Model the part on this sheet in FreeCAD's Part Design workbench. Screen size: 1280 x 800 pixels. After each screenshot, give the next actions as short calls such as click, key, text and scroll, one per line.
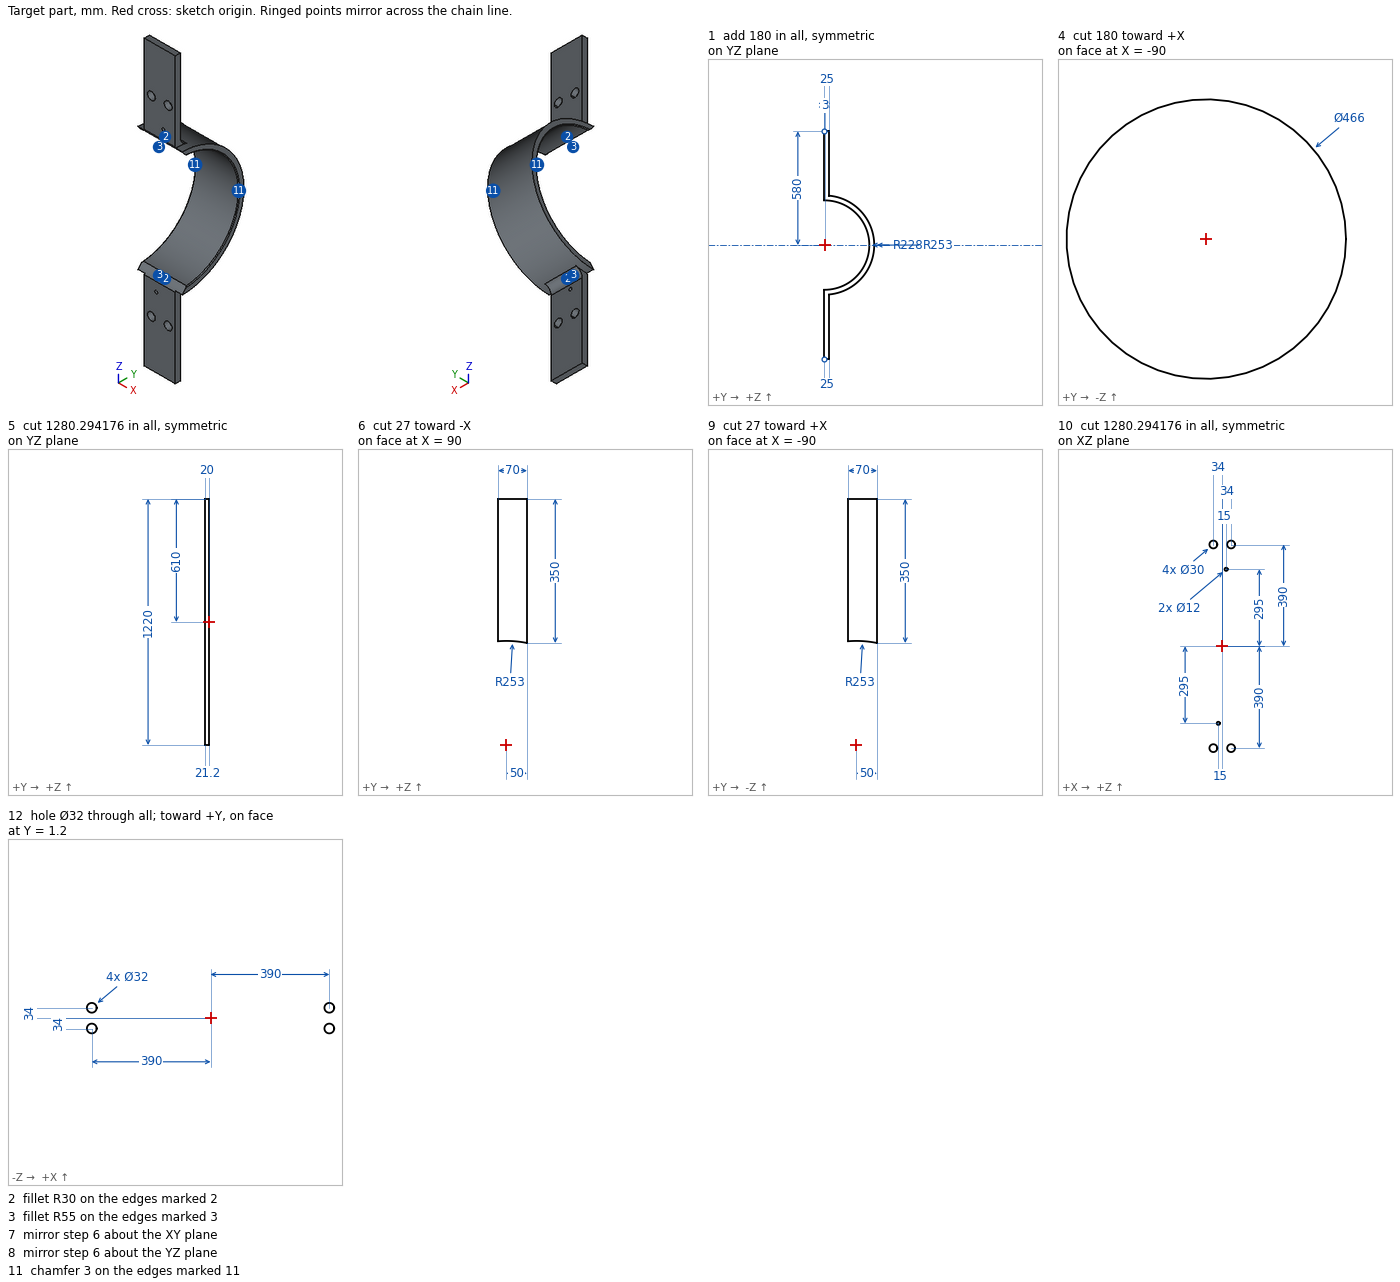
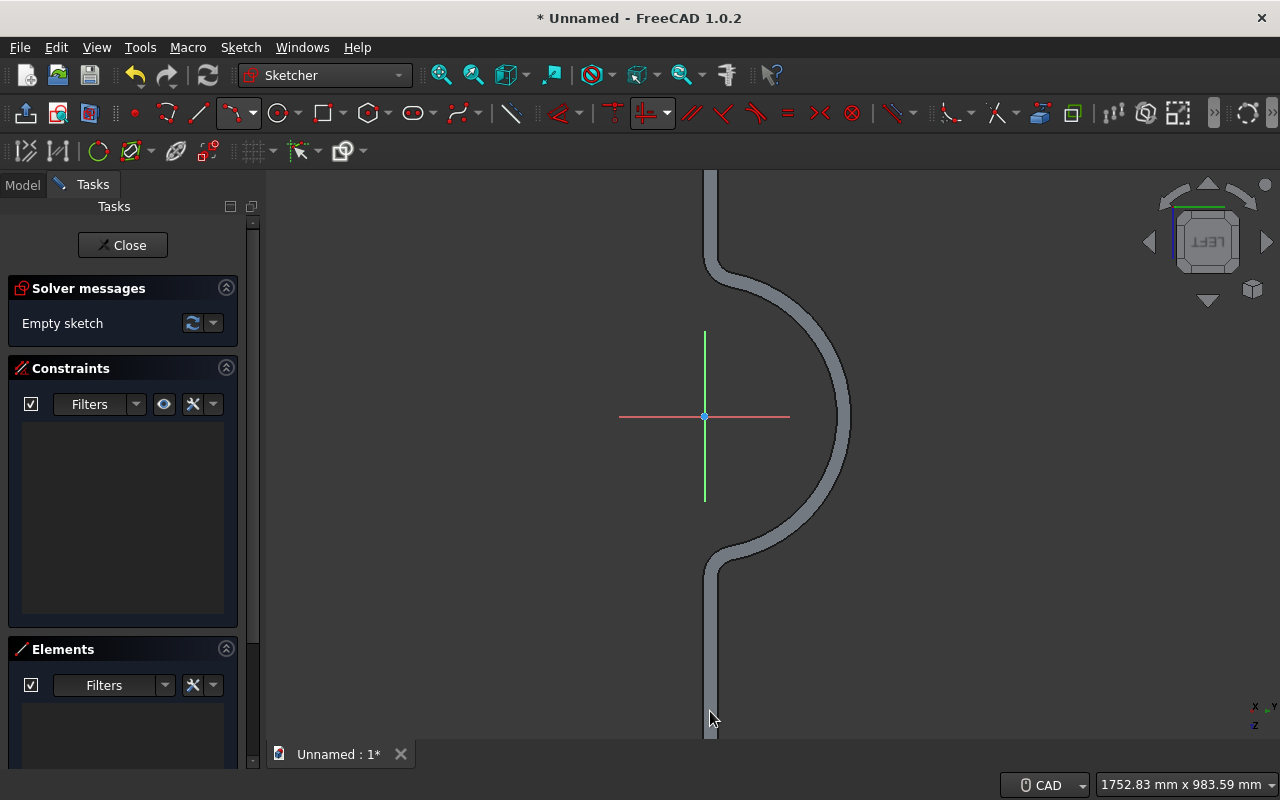
click(278, 114)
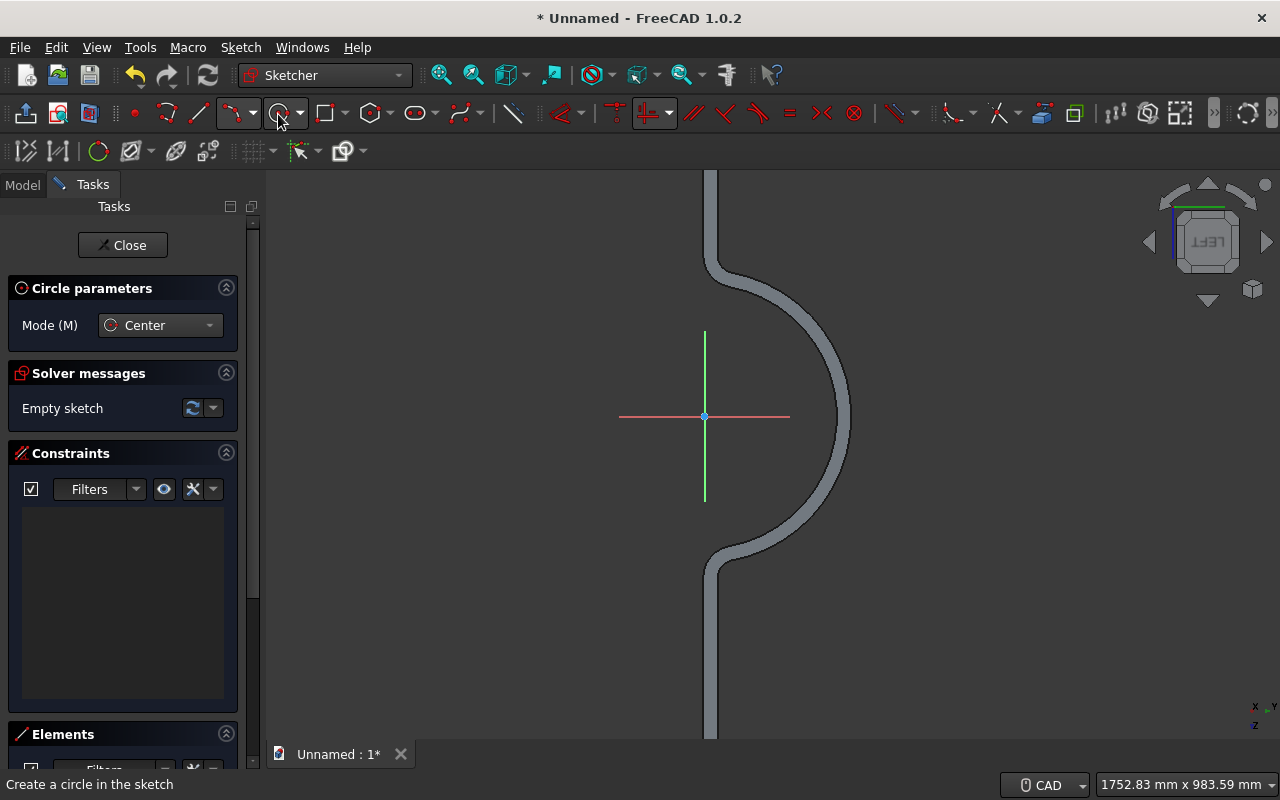
click(705, 417)
move(800, 321)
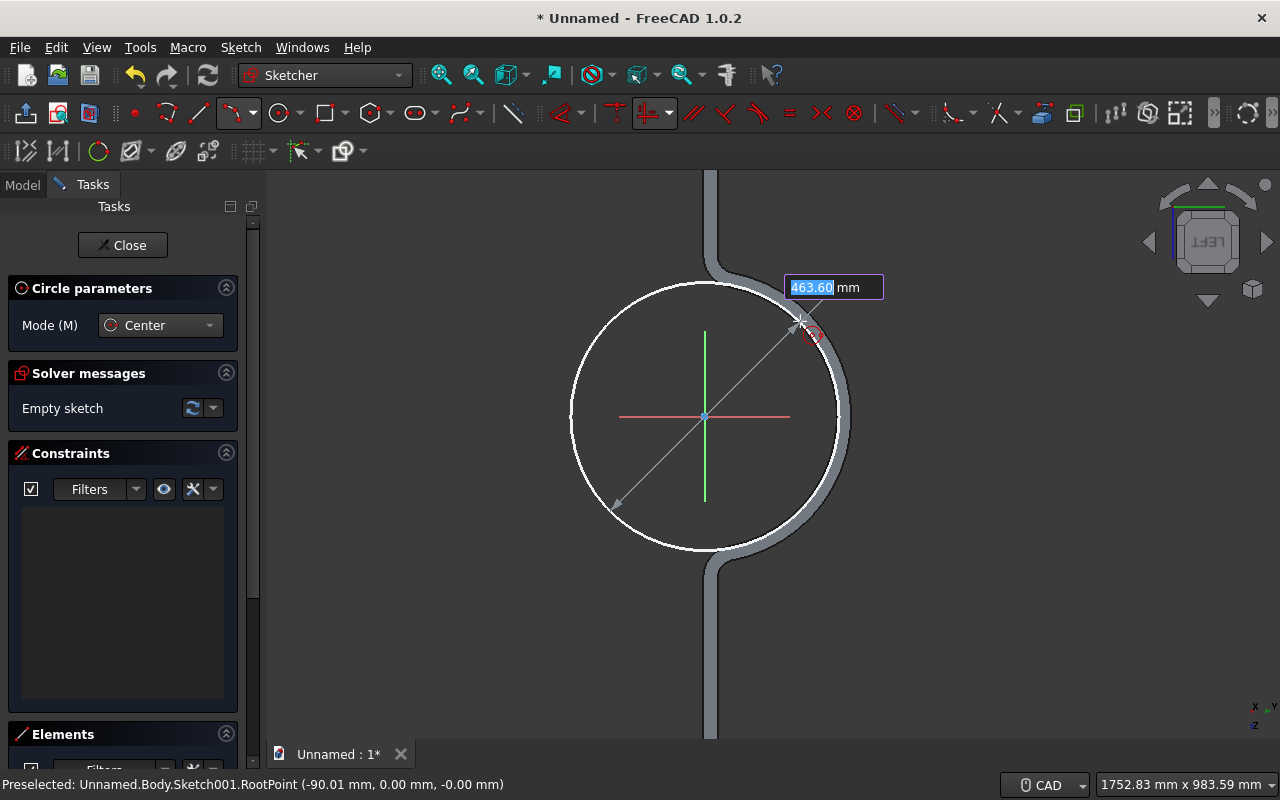
text(466)
key(Return)
key(Escape)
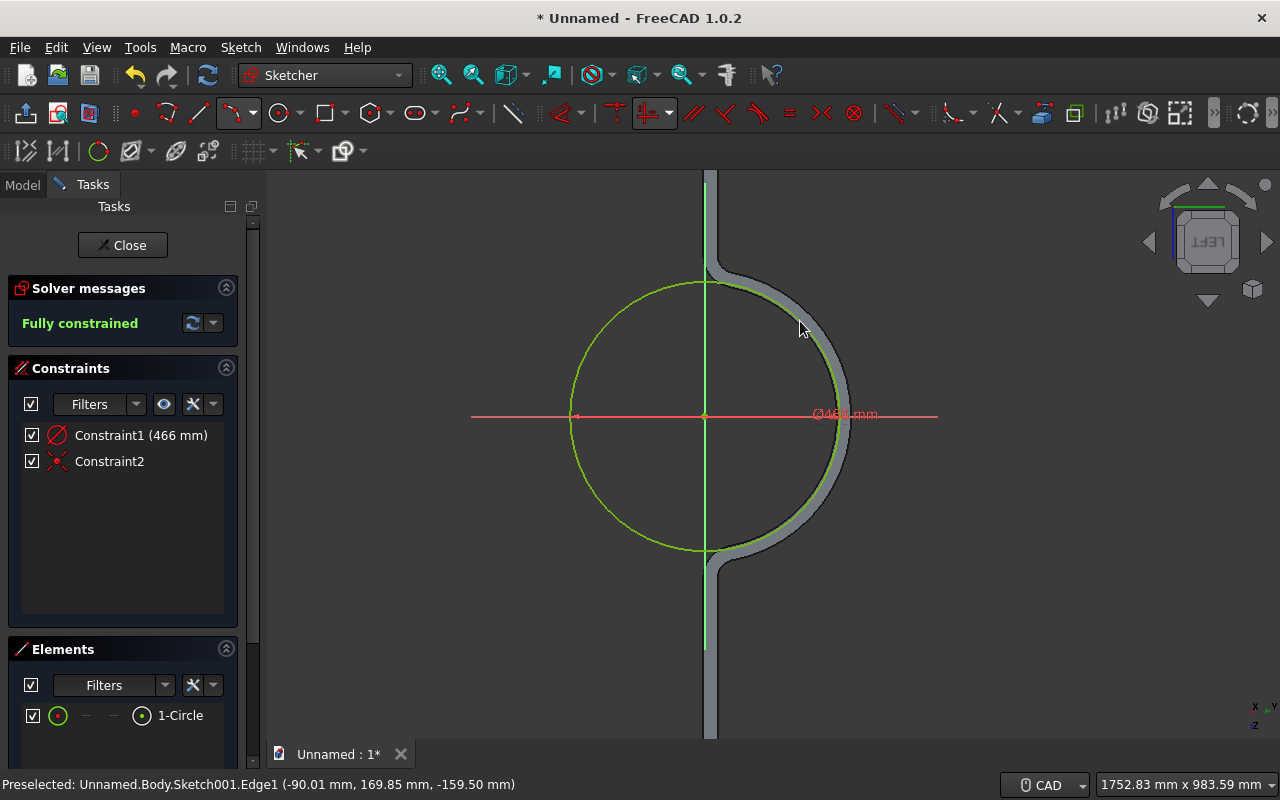
click(123, 245)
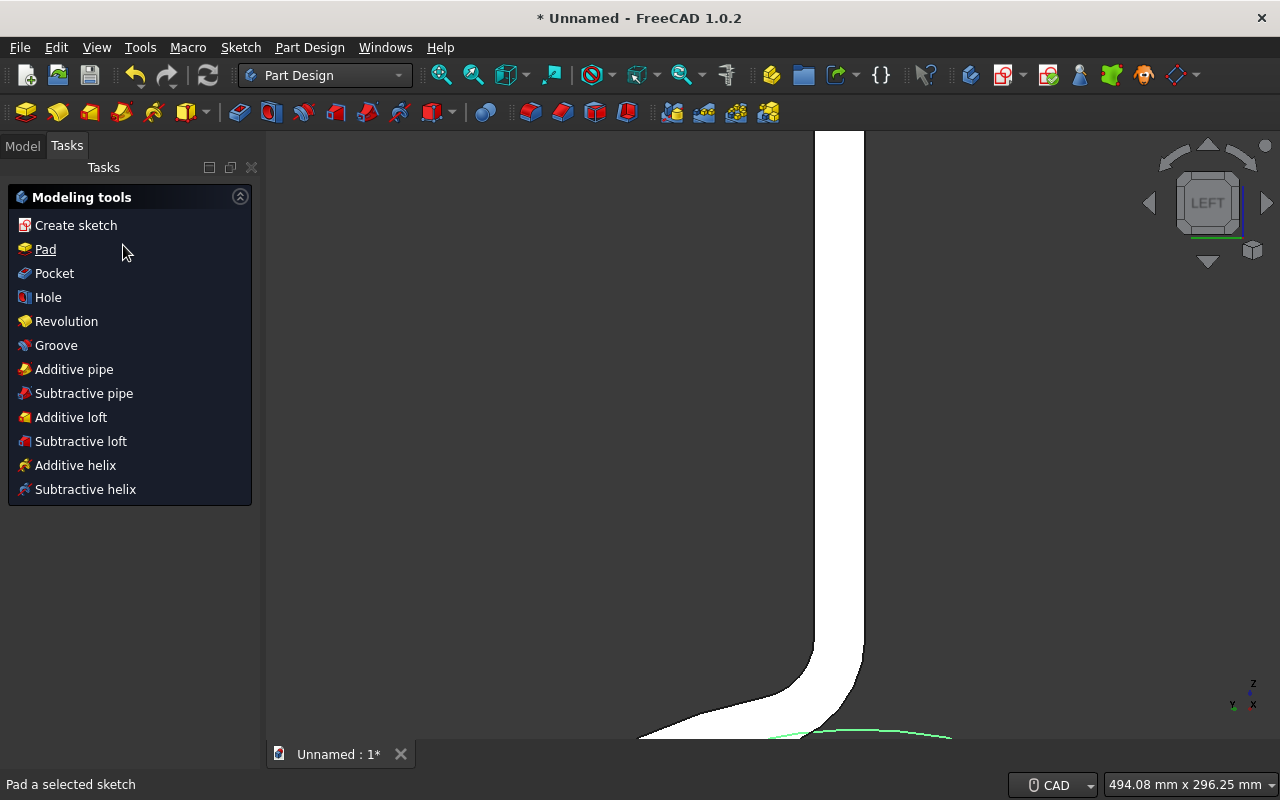
click(240, 112)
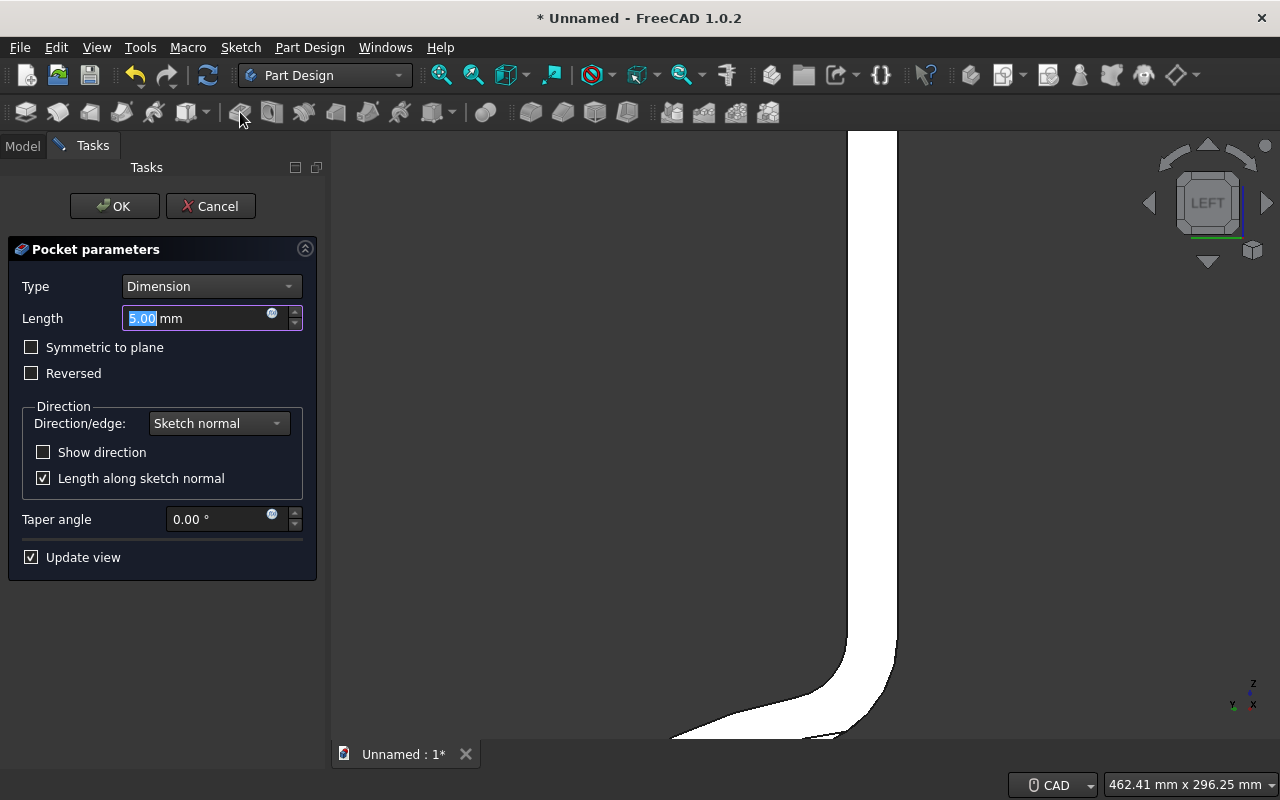
text(180)
key(Tab)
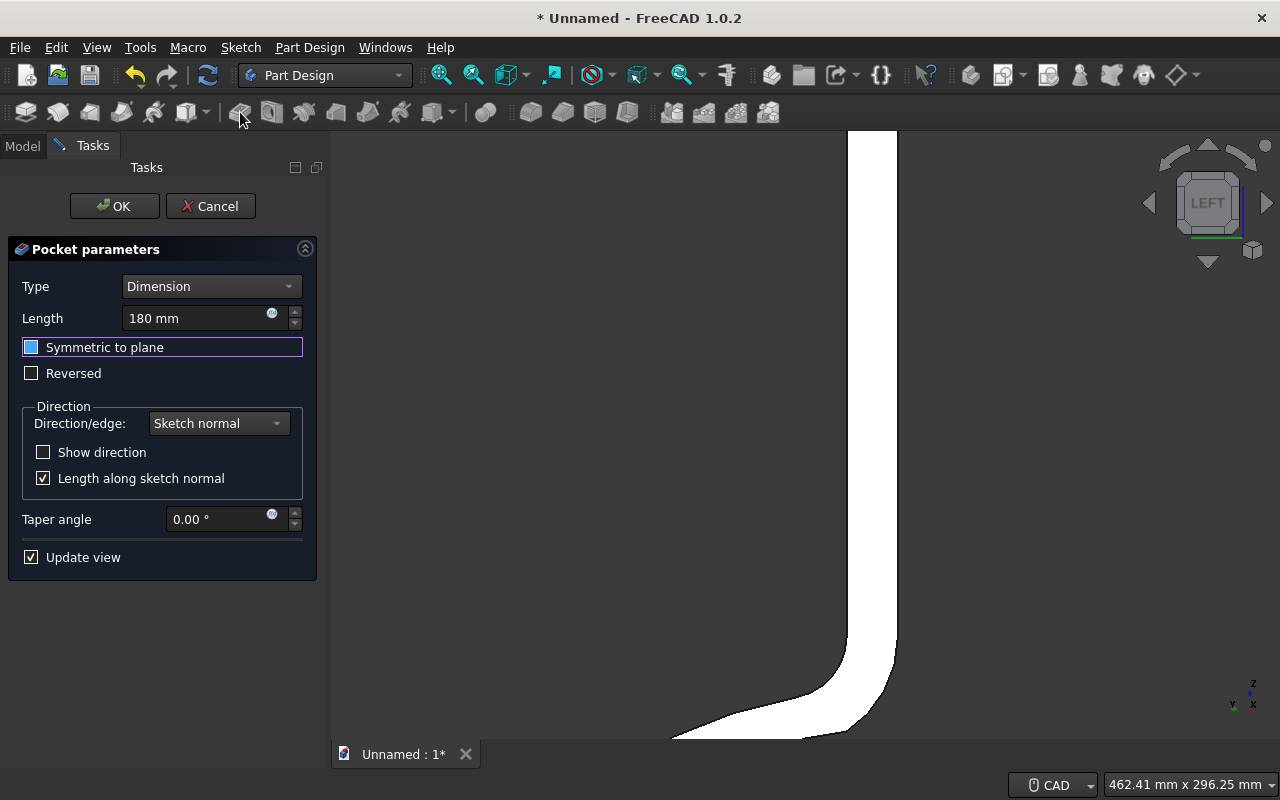
click(115, 206)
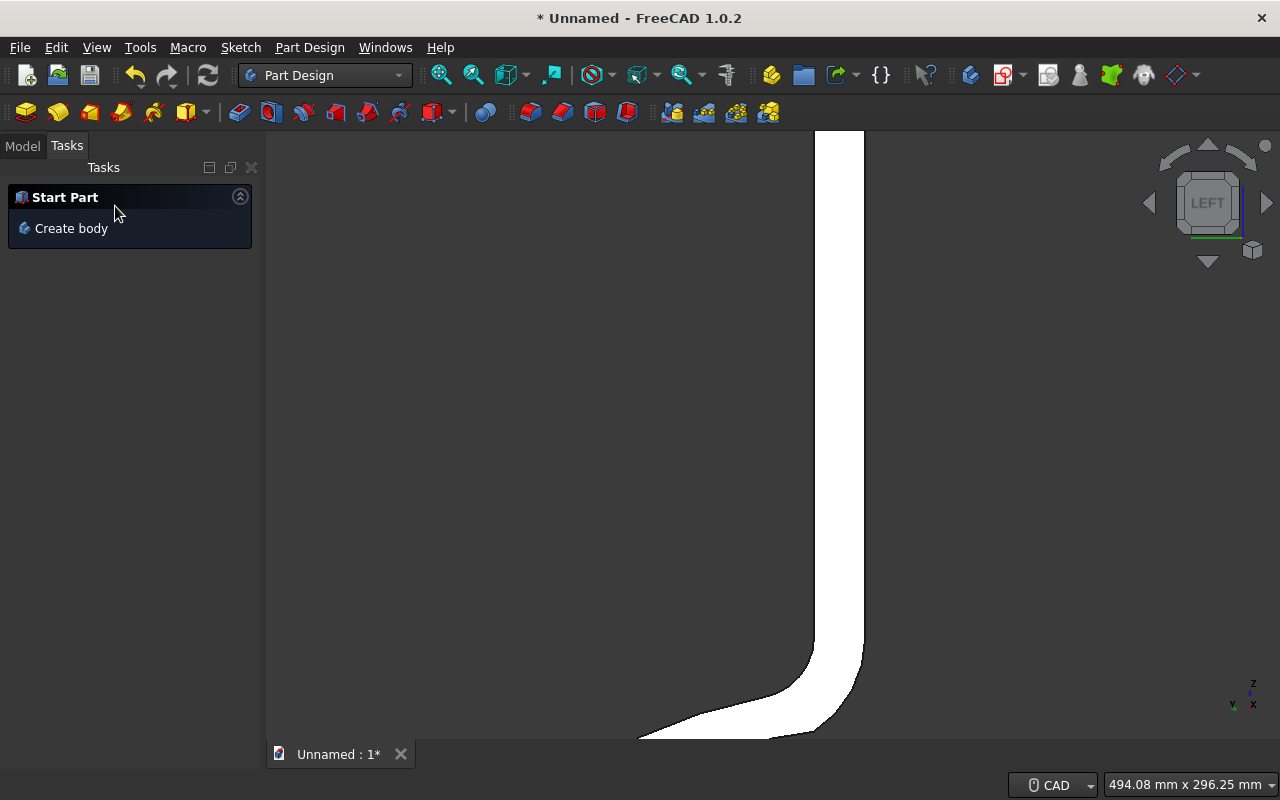
click(442, 76)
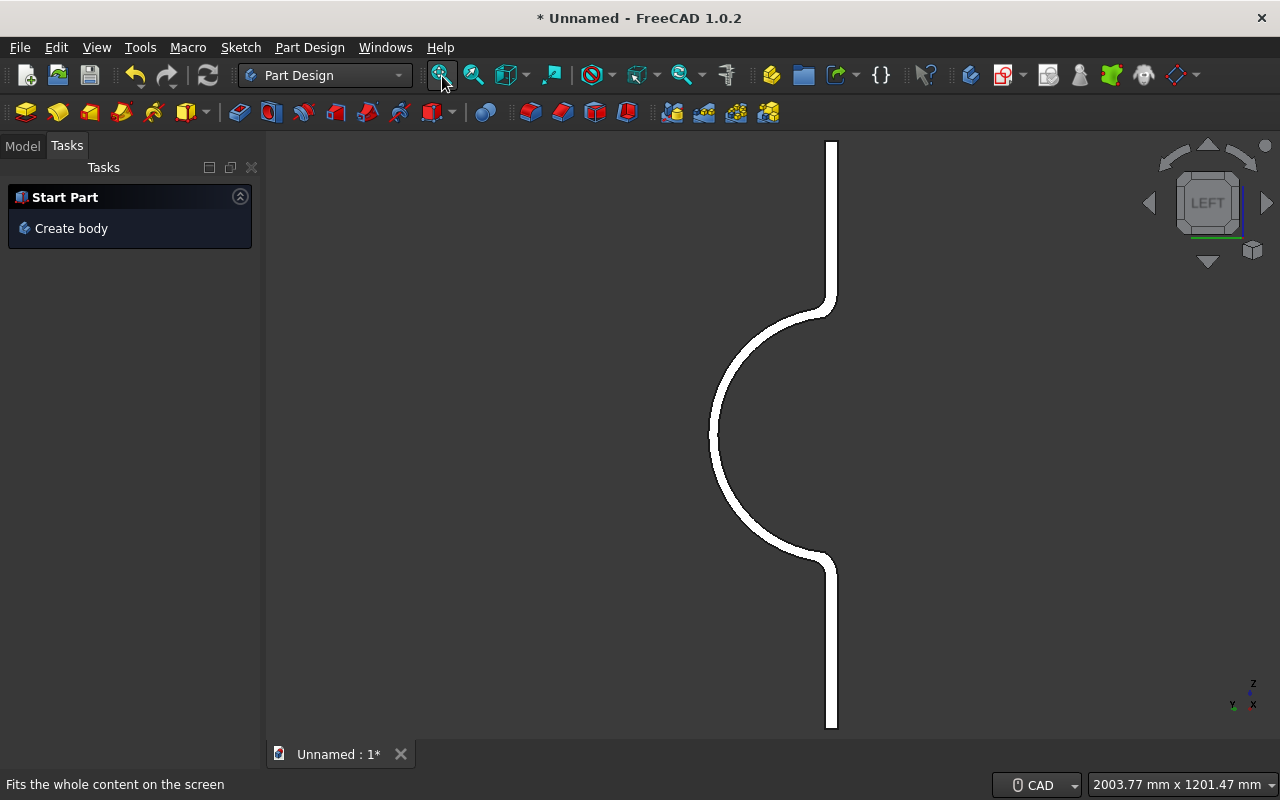
click(1004, 76)